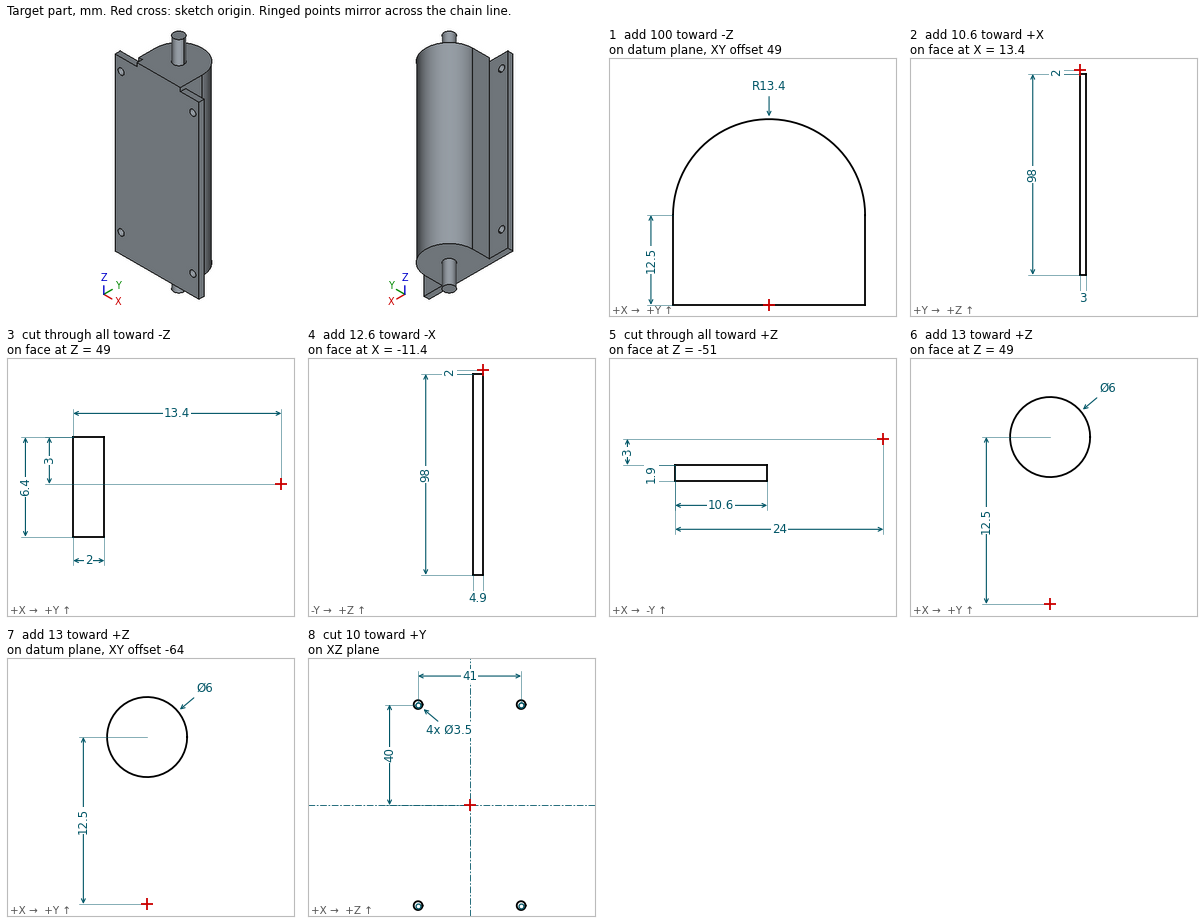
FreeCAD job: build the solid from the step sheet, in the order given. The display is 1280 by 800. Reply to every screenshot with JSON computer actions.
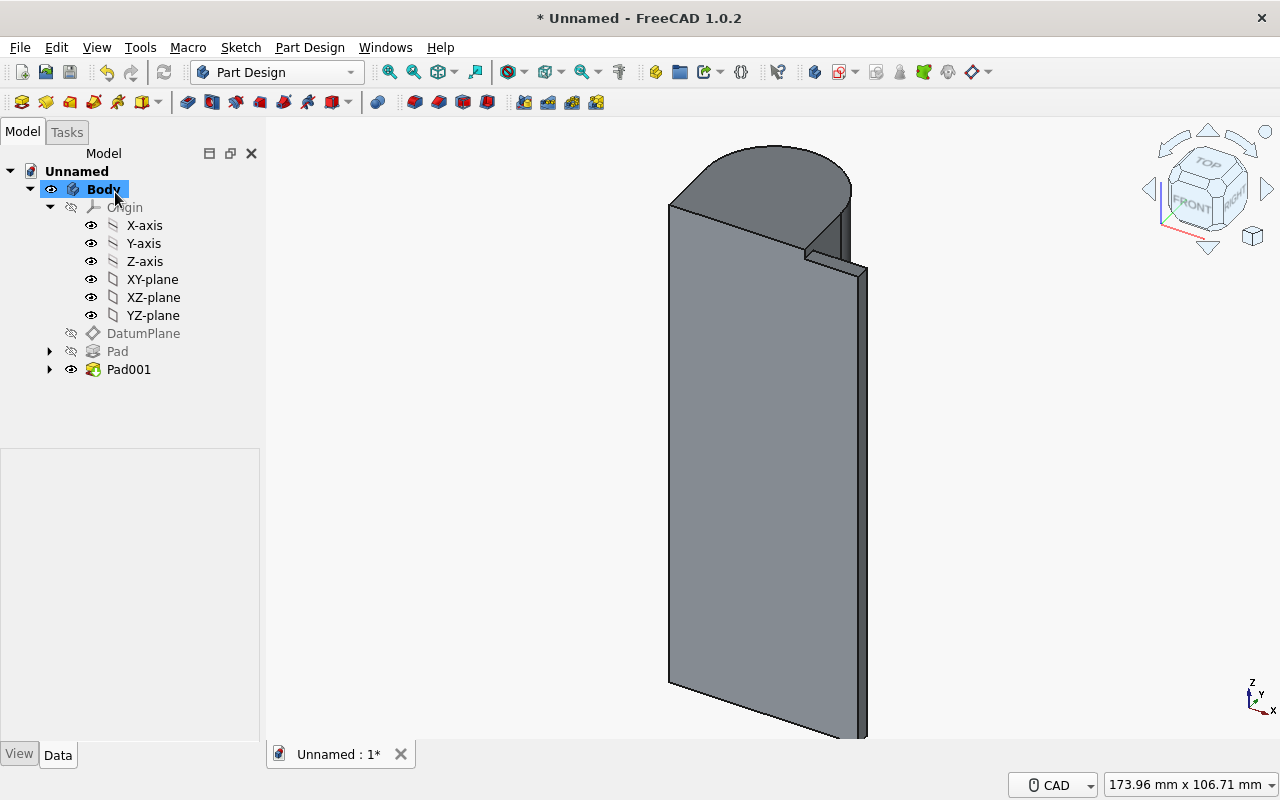
{"action": "left_click", "coordinate": [390, 72]}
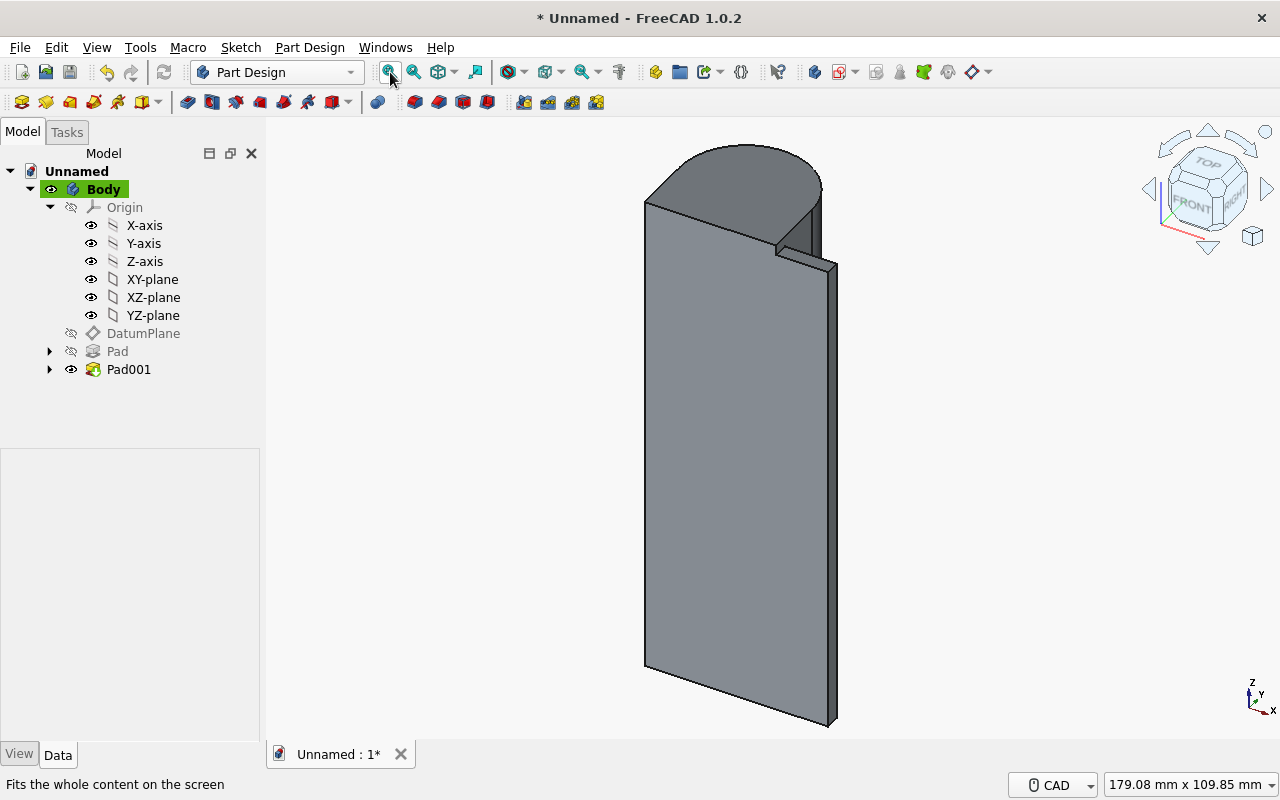
{"action": "left_click", "coordinate": [747, 186]}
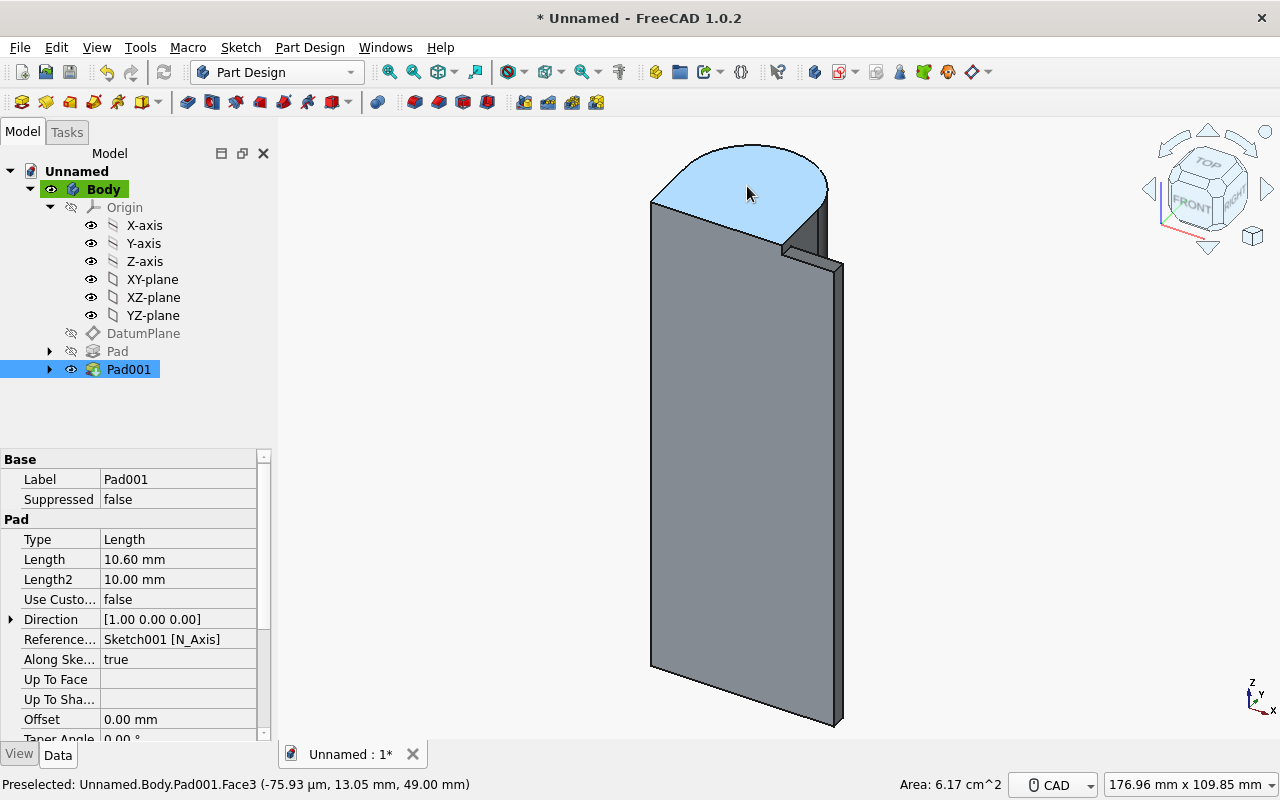
{"action": "left_click", "coordinate": [840, 72]}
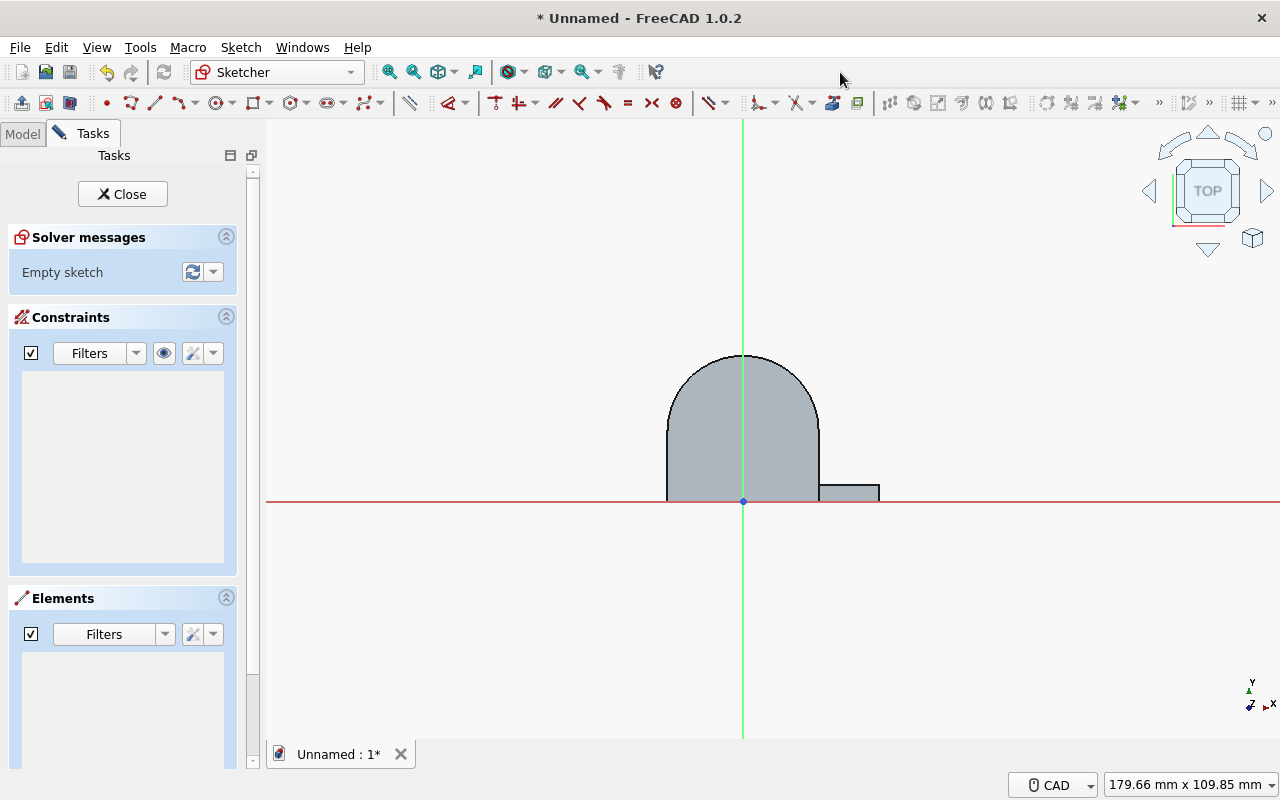
{"action": "scroll", "coordinate": [705, 515], "scroll_direction": "up", "scroll_amount": 10}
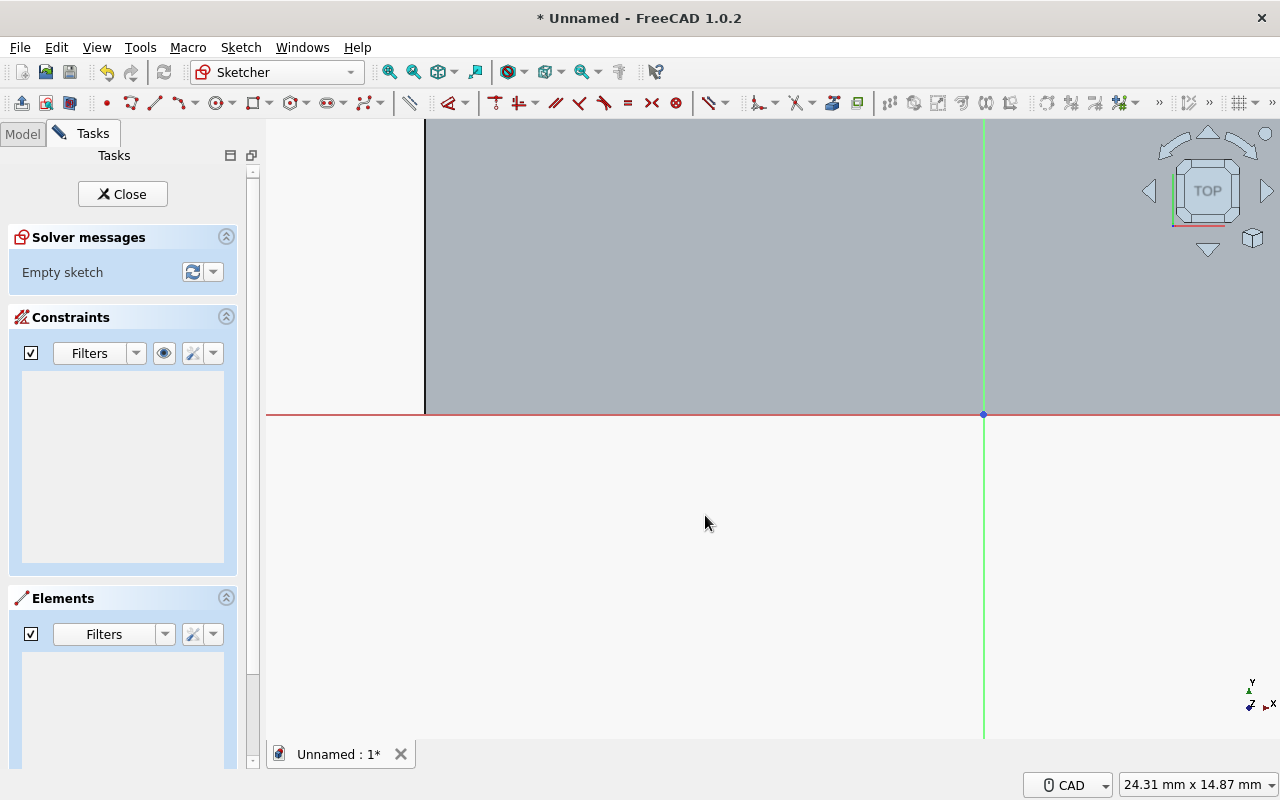
{"action": "left_click", "coordinate": [254, 104]}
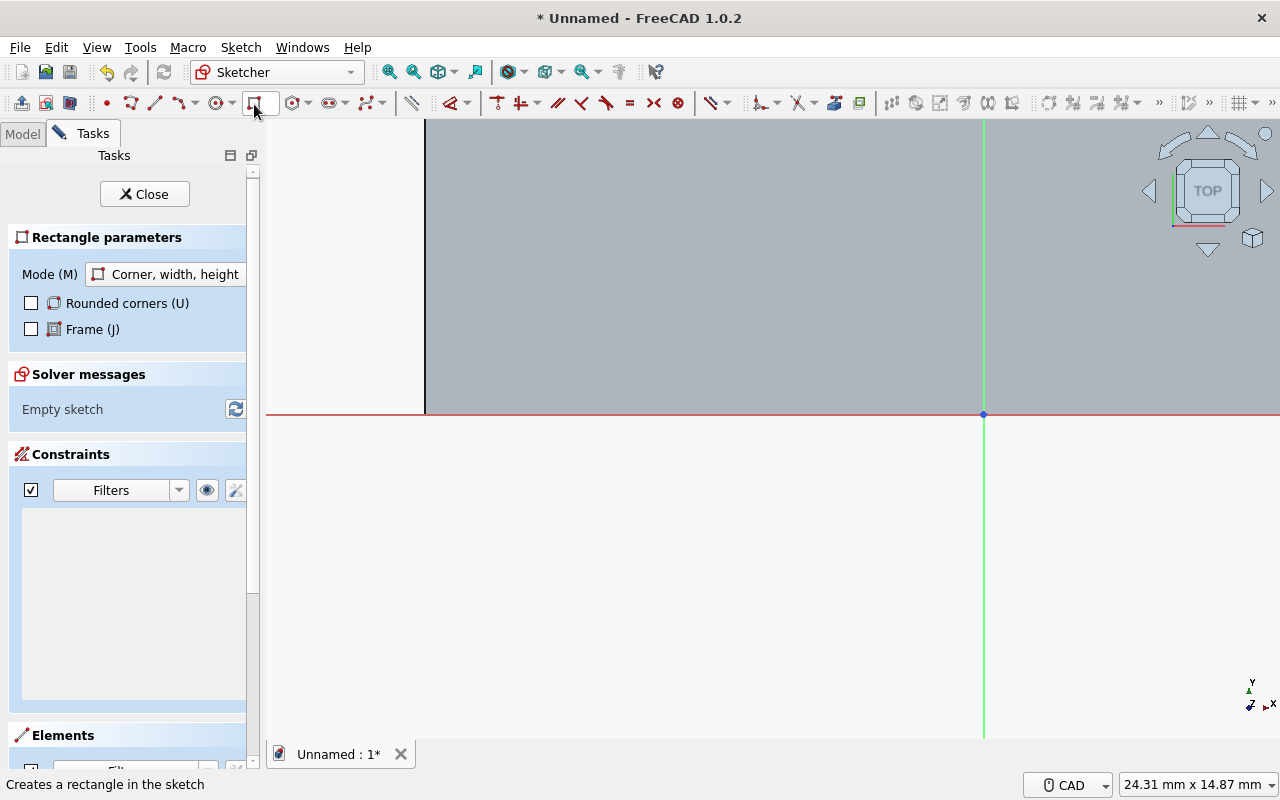
{"action": "left_click", "coordinate": [425, 289]}
{"action": "left_click", "coordinate": [508, 556]}
{"action": "key", "text": "Escape"}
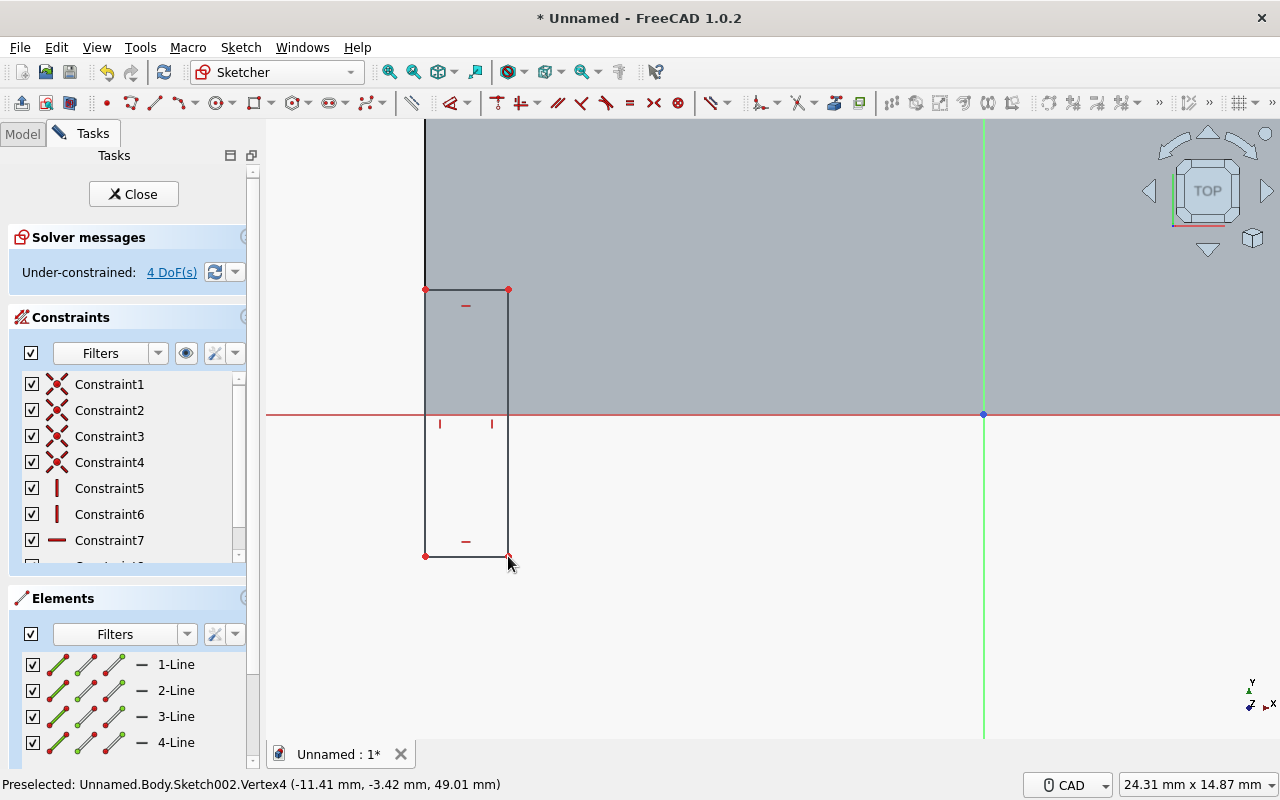
{"action": "left_click", "coordinate": [450, 104]}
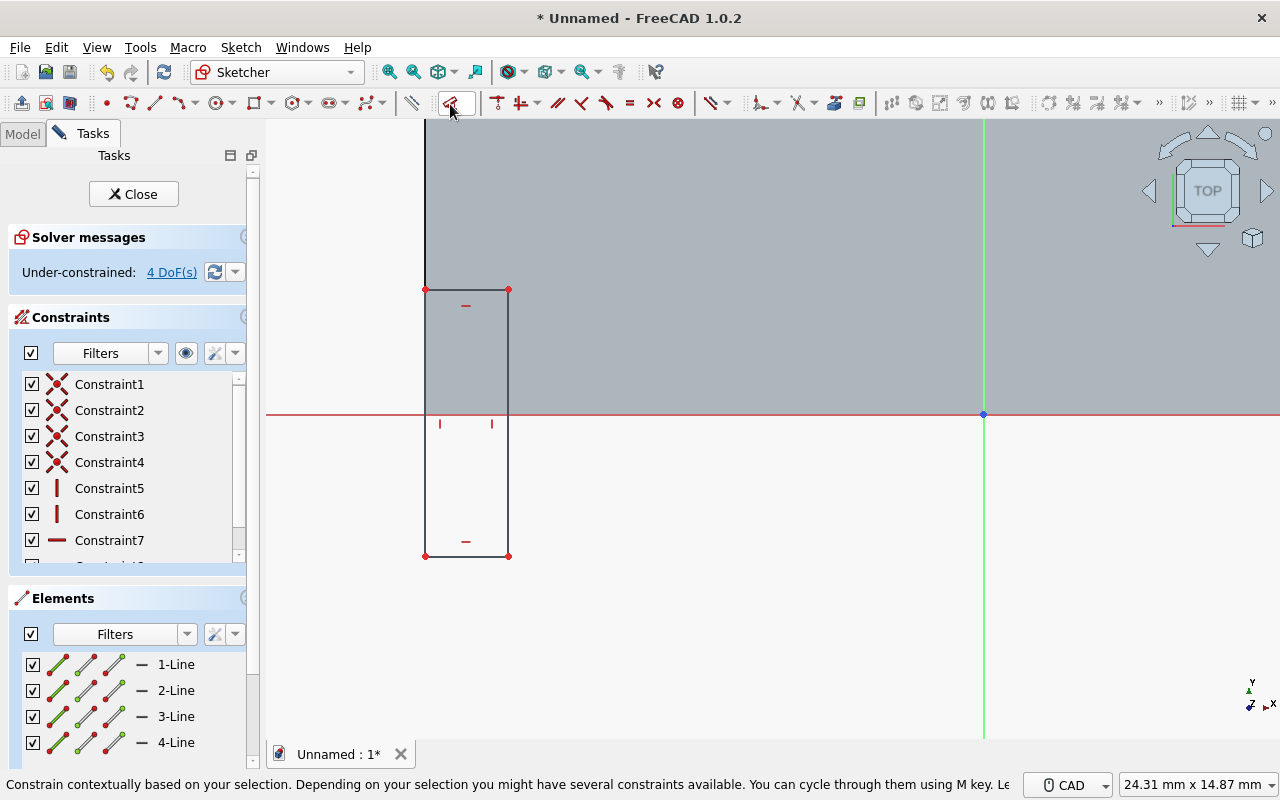
{"action": "left_click", "coordinate": [450, 557]}
{"action": "left_click", "coordinate": [467, 591]}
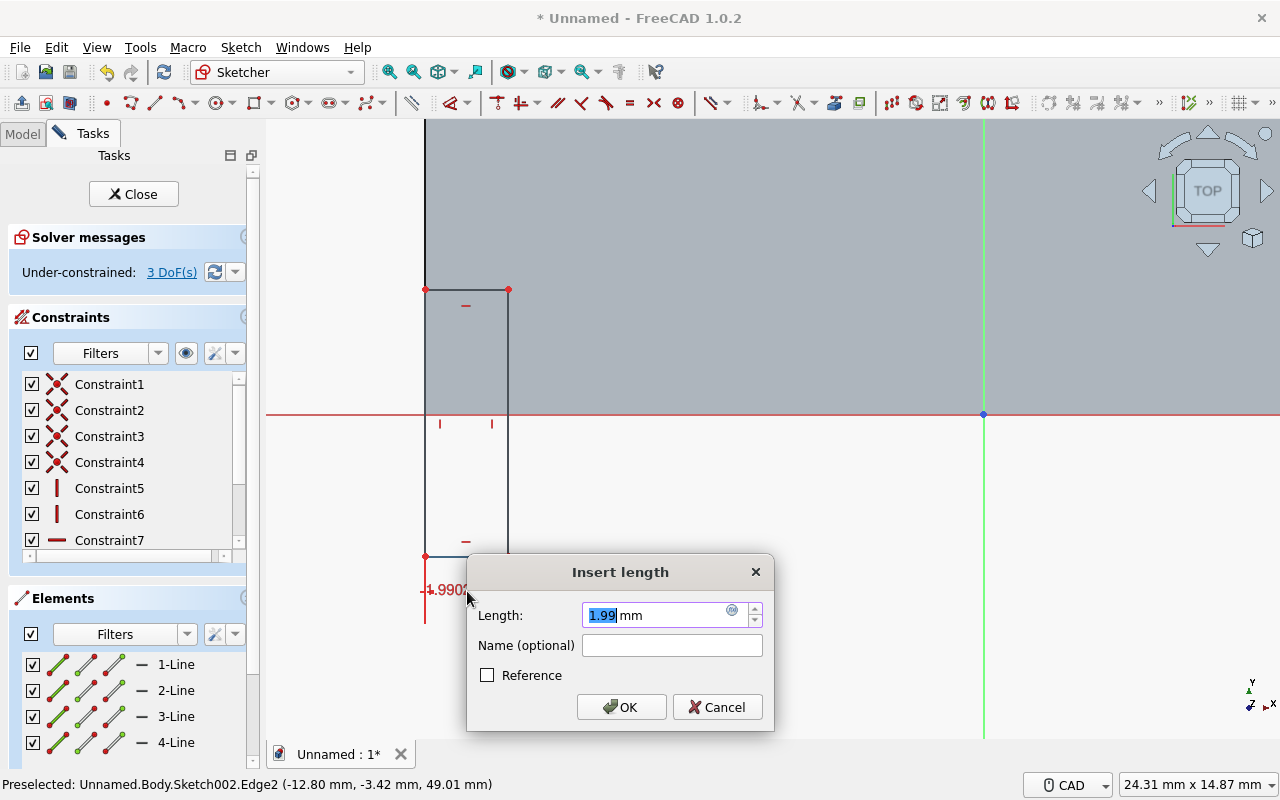
{"action": "type", "text": "2"}
{"action": "key", "text": "Return"}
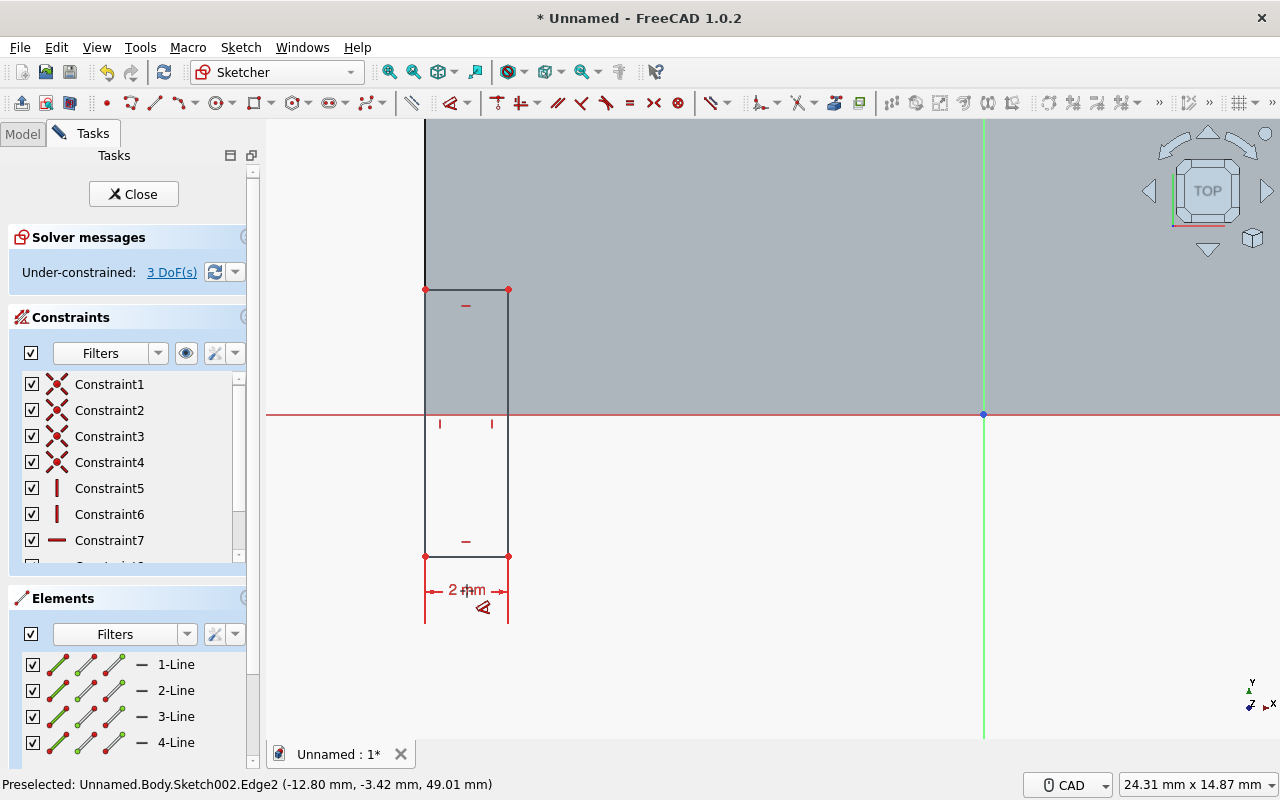
{"action": "left_click", "coordinate": [425, 290]}
{"action": "left_click", "coordinate": [1018, 352]}